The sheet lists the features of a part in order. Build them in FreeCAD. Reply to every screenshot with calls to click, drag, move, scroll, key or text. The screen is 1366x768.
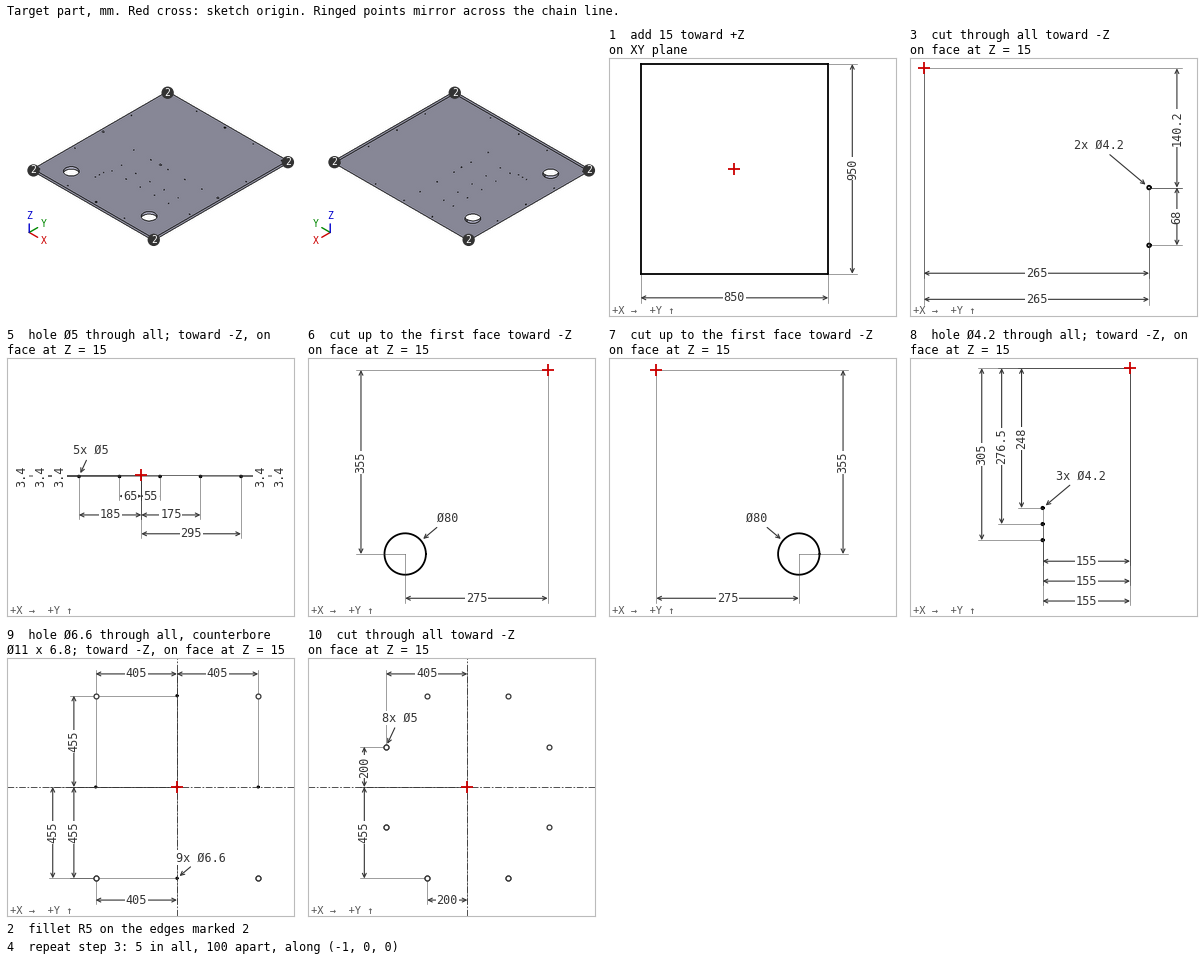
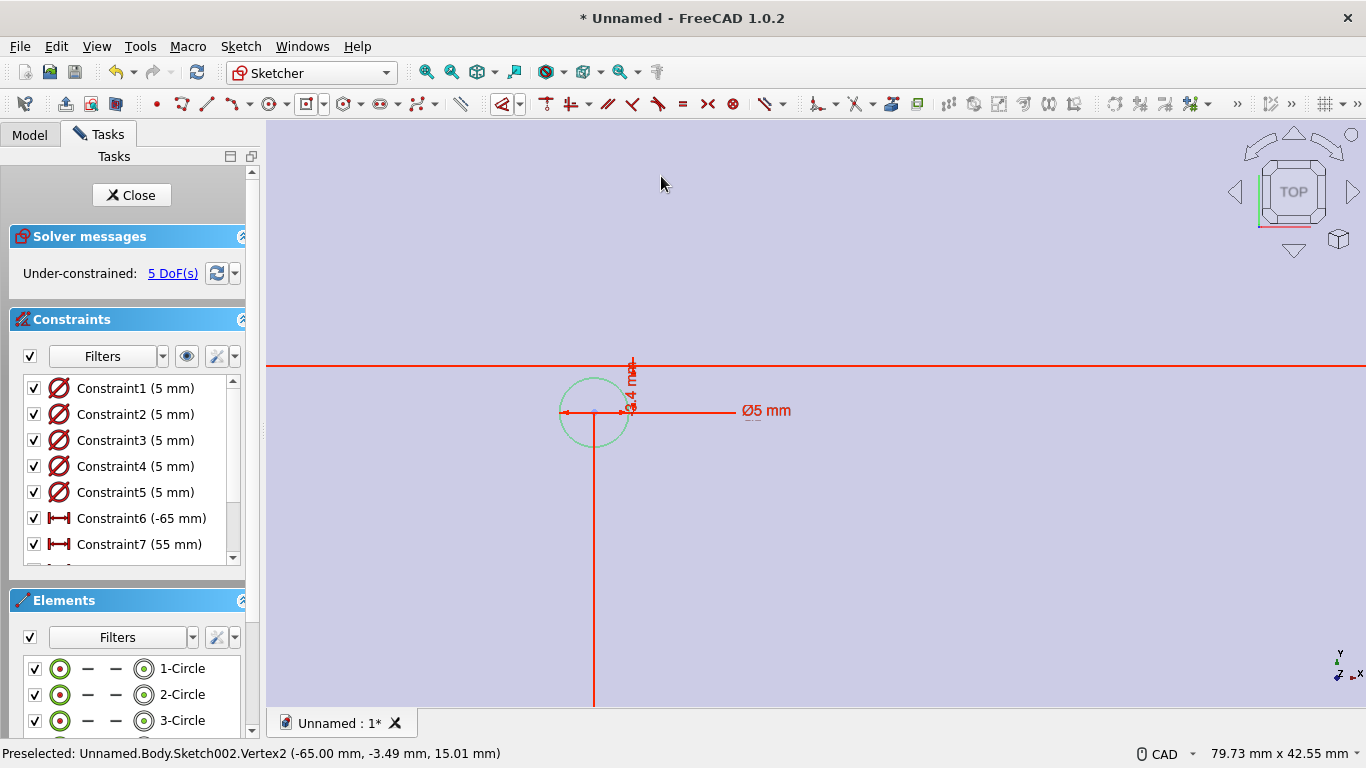
scroll(598, 414, down, 12)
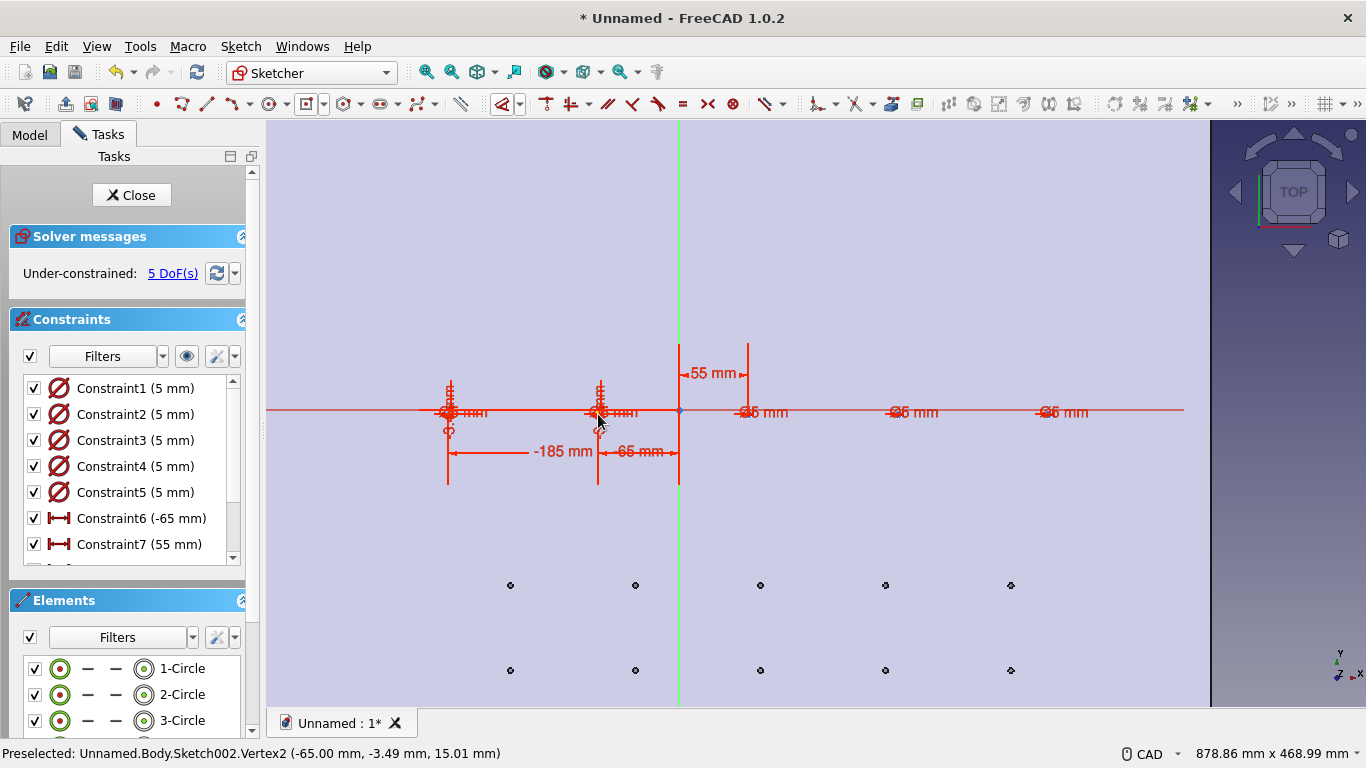
scroll(748, 414, up, 12)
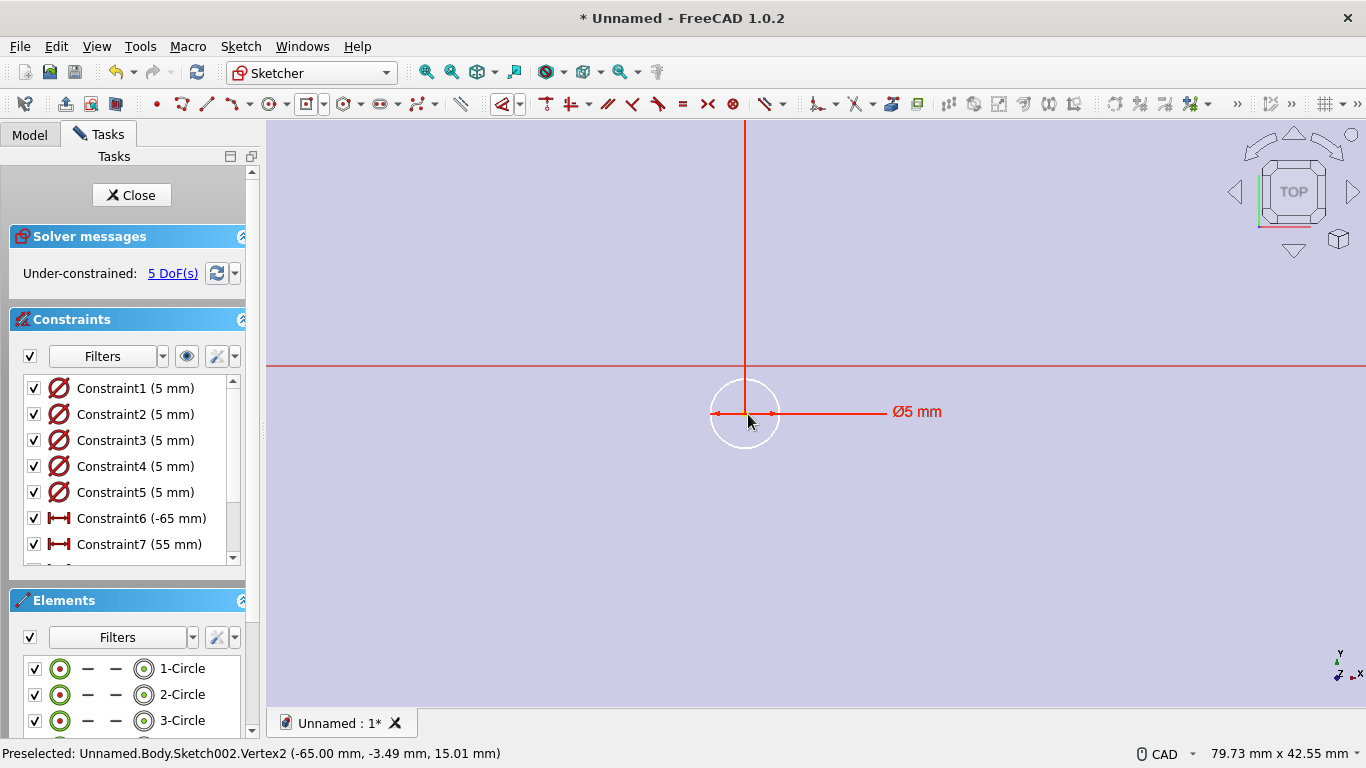
click(745, 414)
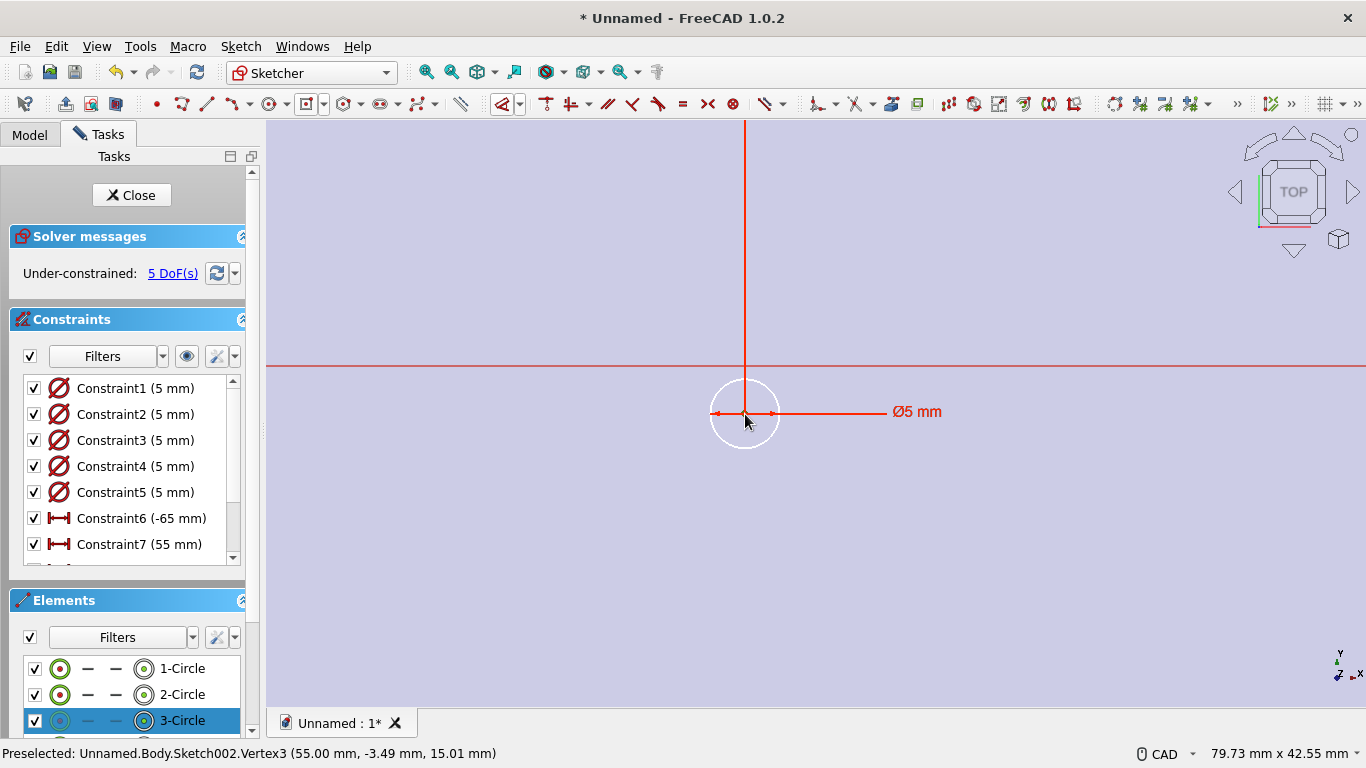
key(i)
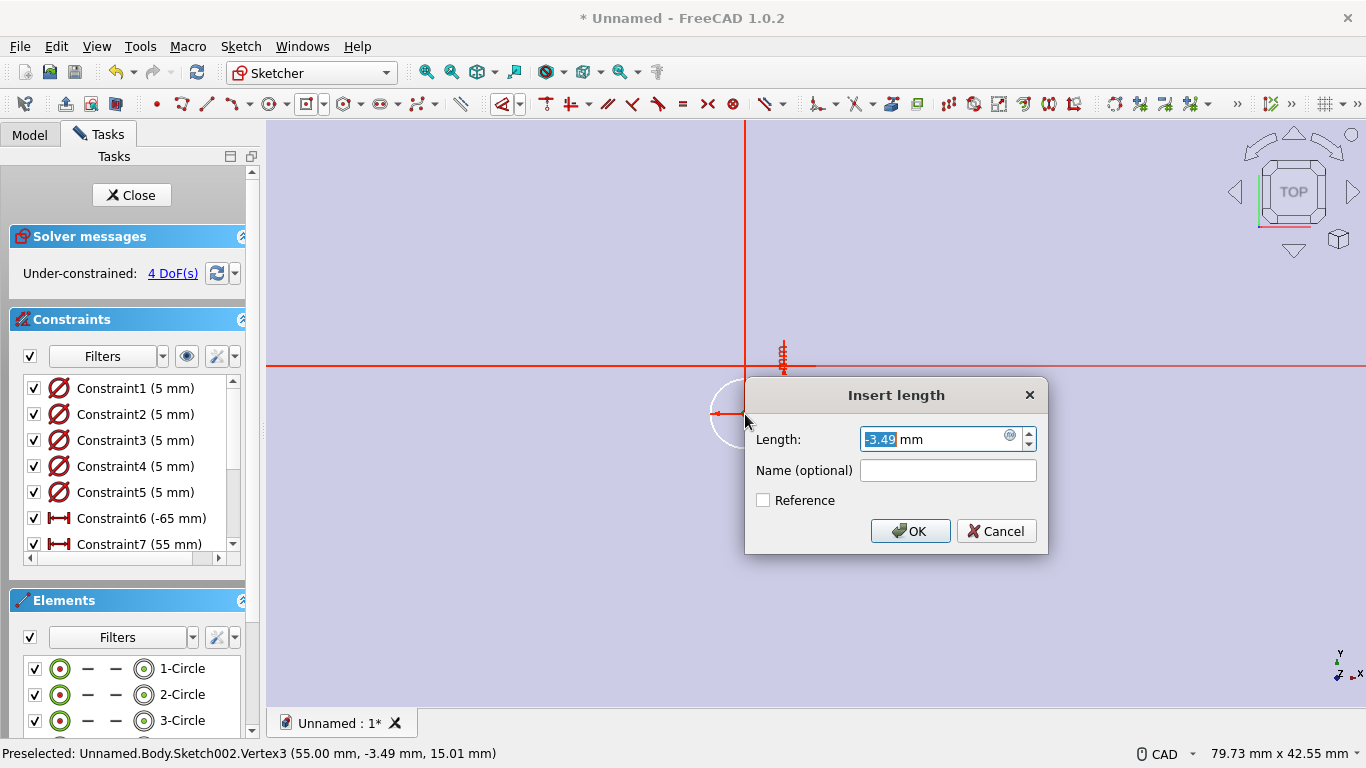
text(-3.4)
key(Return)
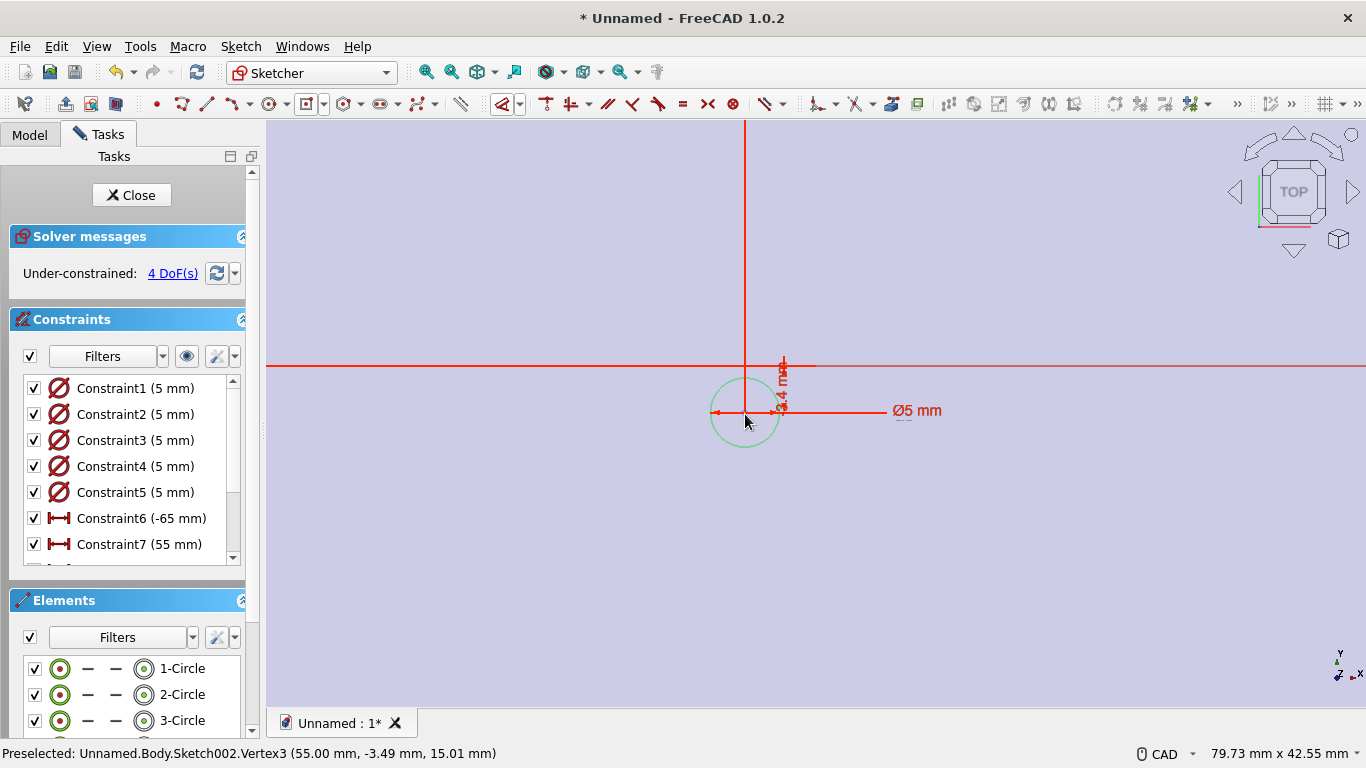
scroll(748, 414, down, 12)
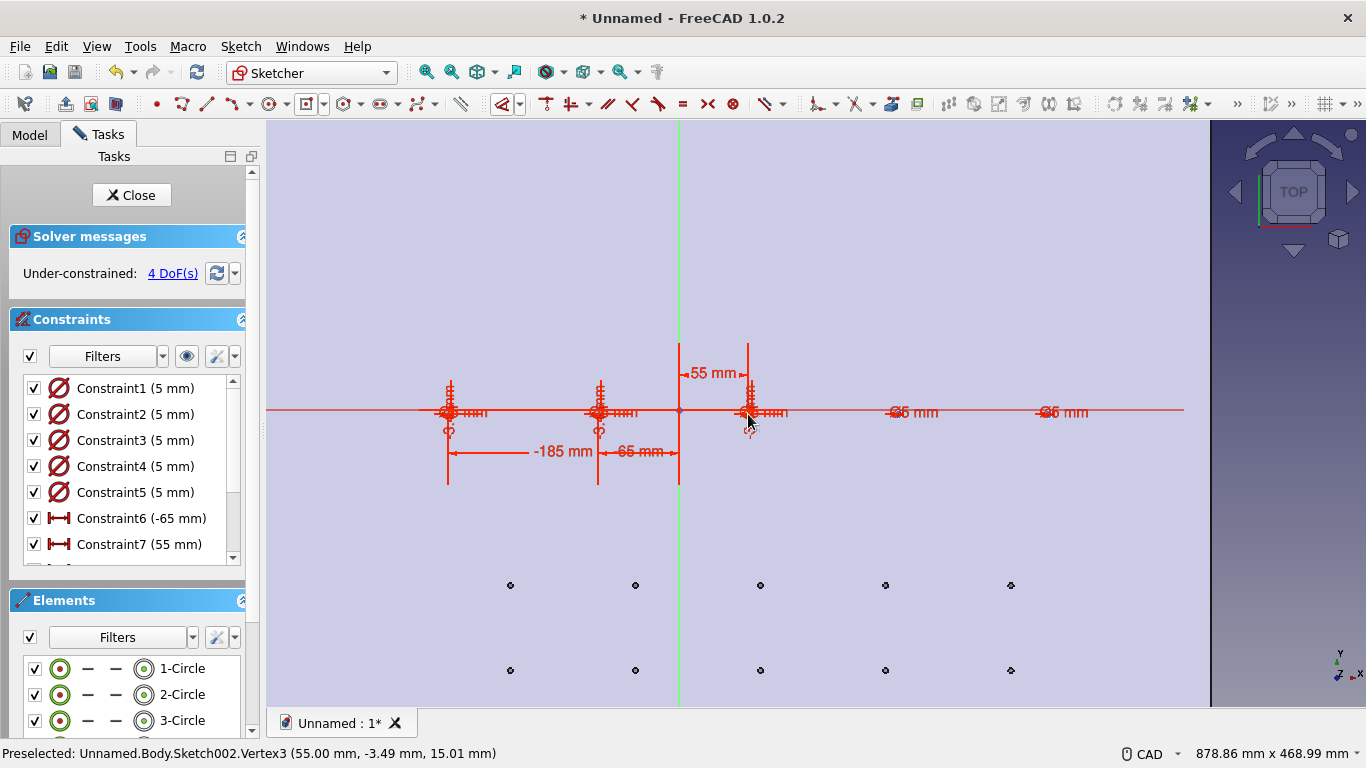
click(898, 414)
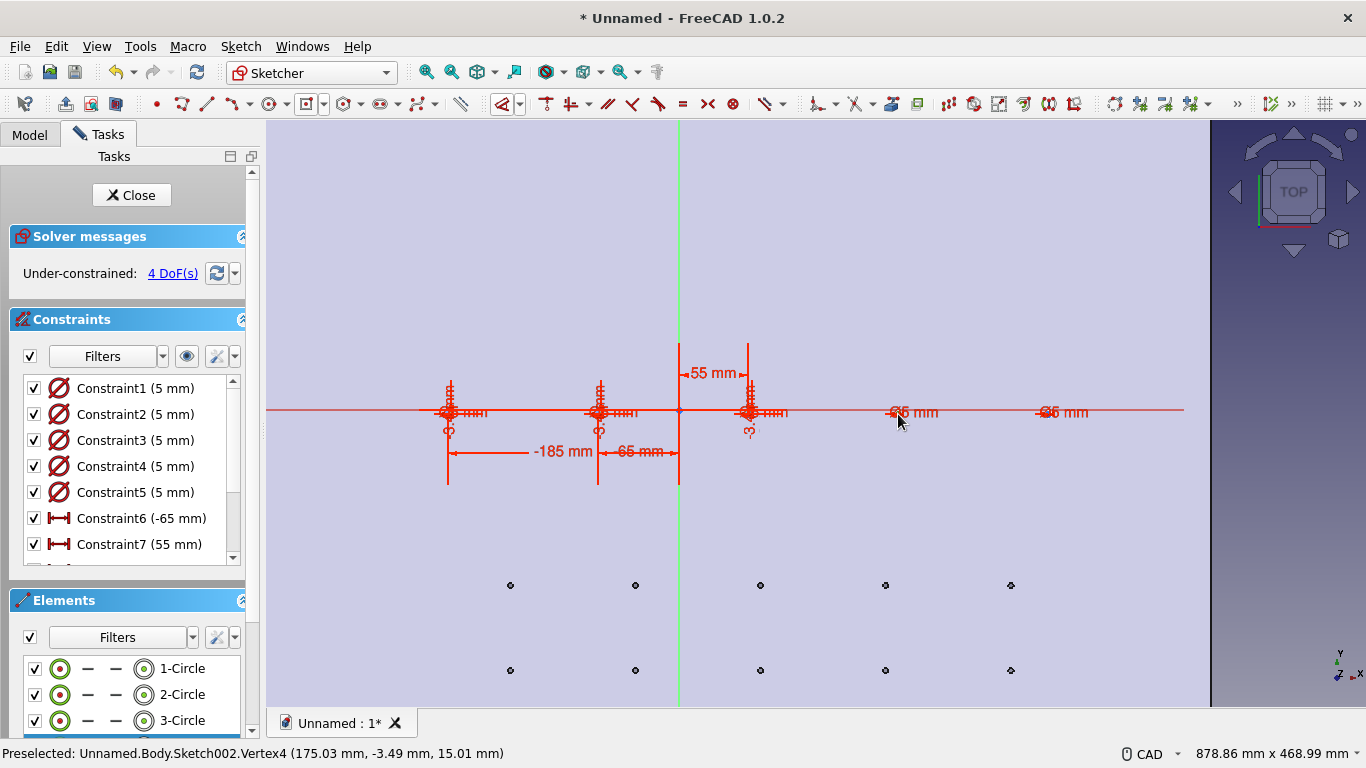
click(520, 104)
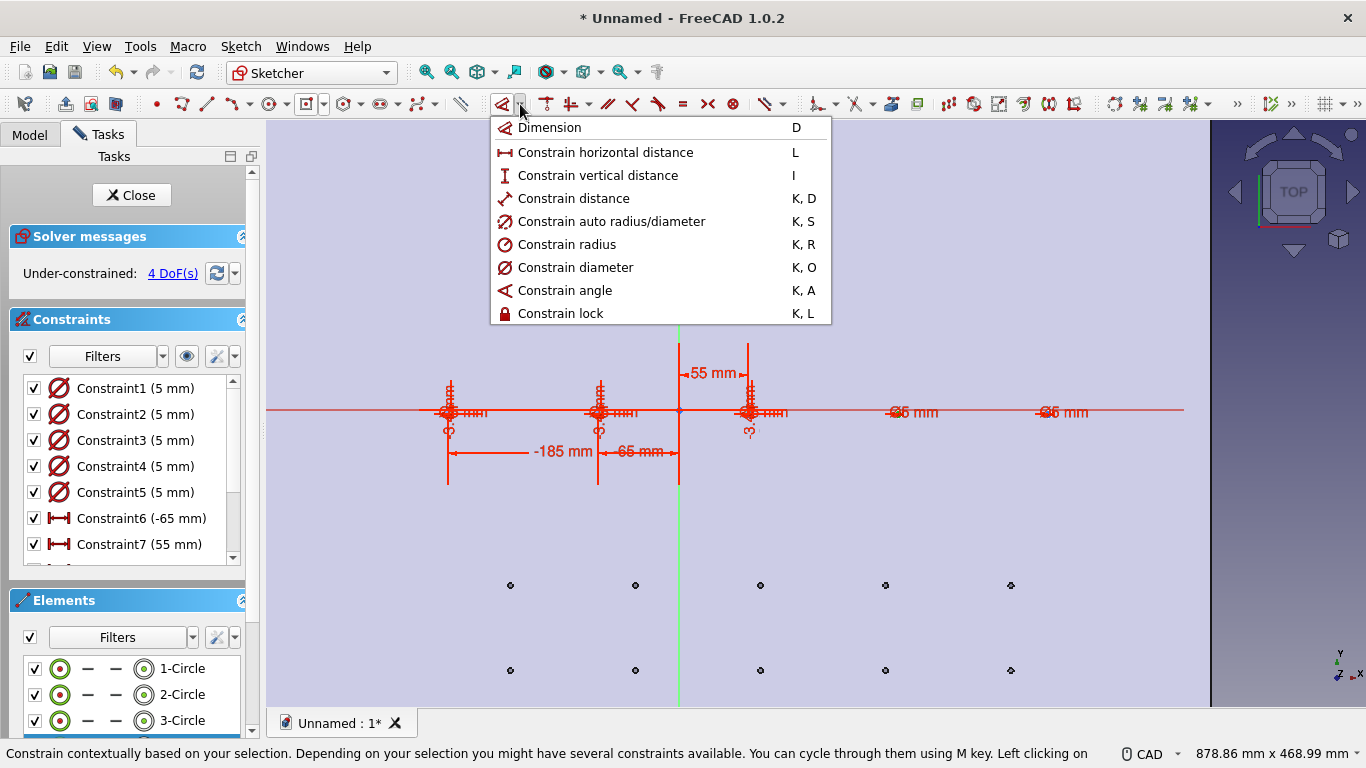
click(661, 152)